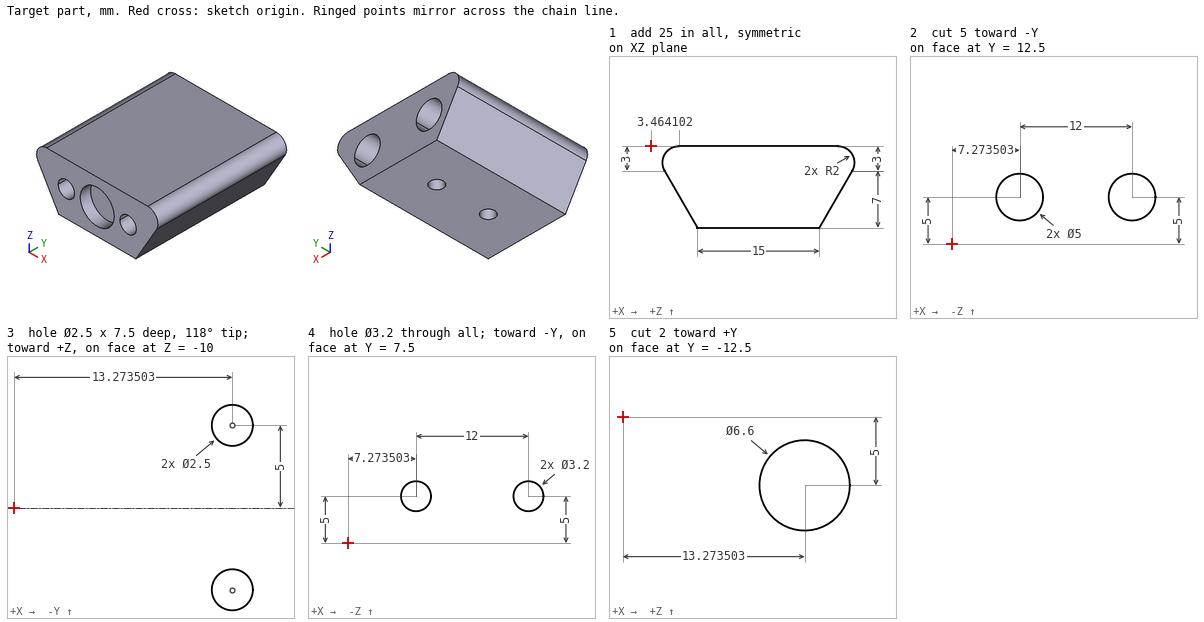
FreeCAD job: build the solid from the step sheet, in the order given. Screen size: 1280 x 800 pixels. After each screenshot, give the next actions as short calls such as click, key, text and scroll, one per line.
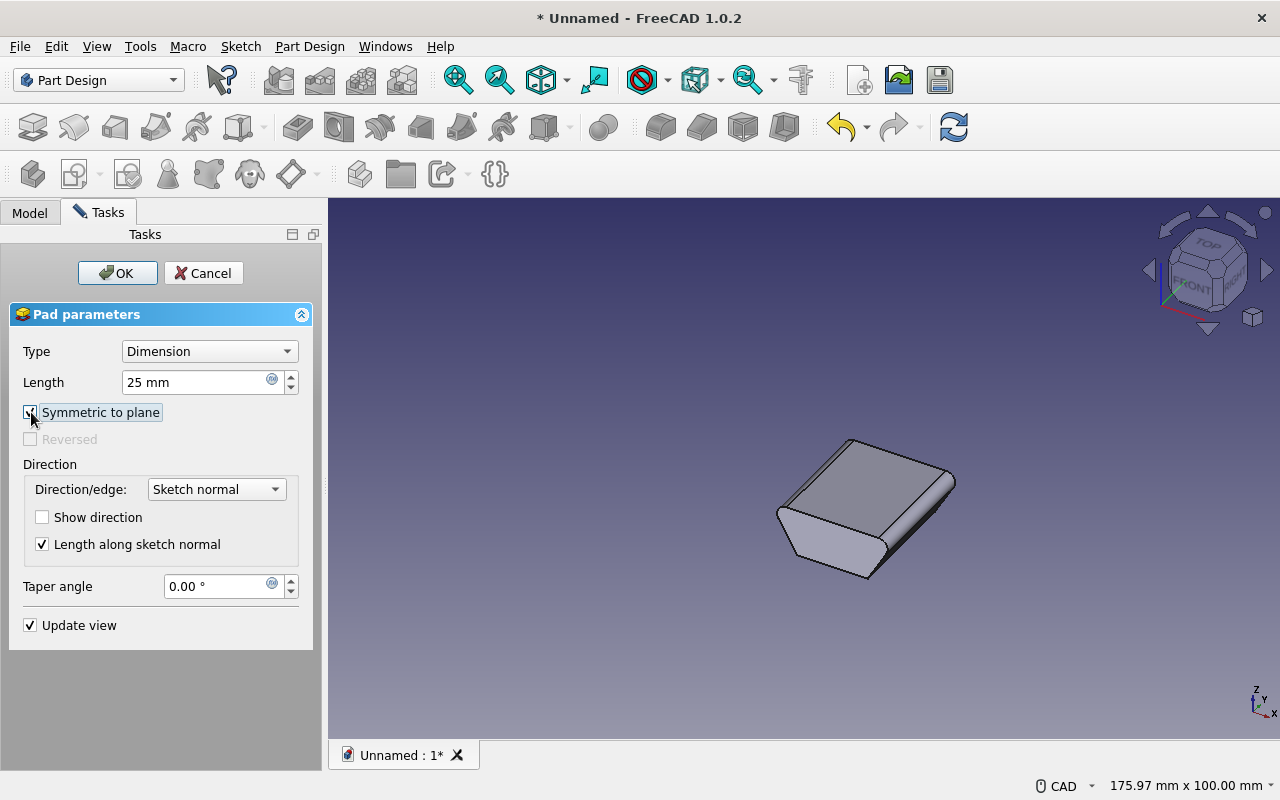
click(118, 273)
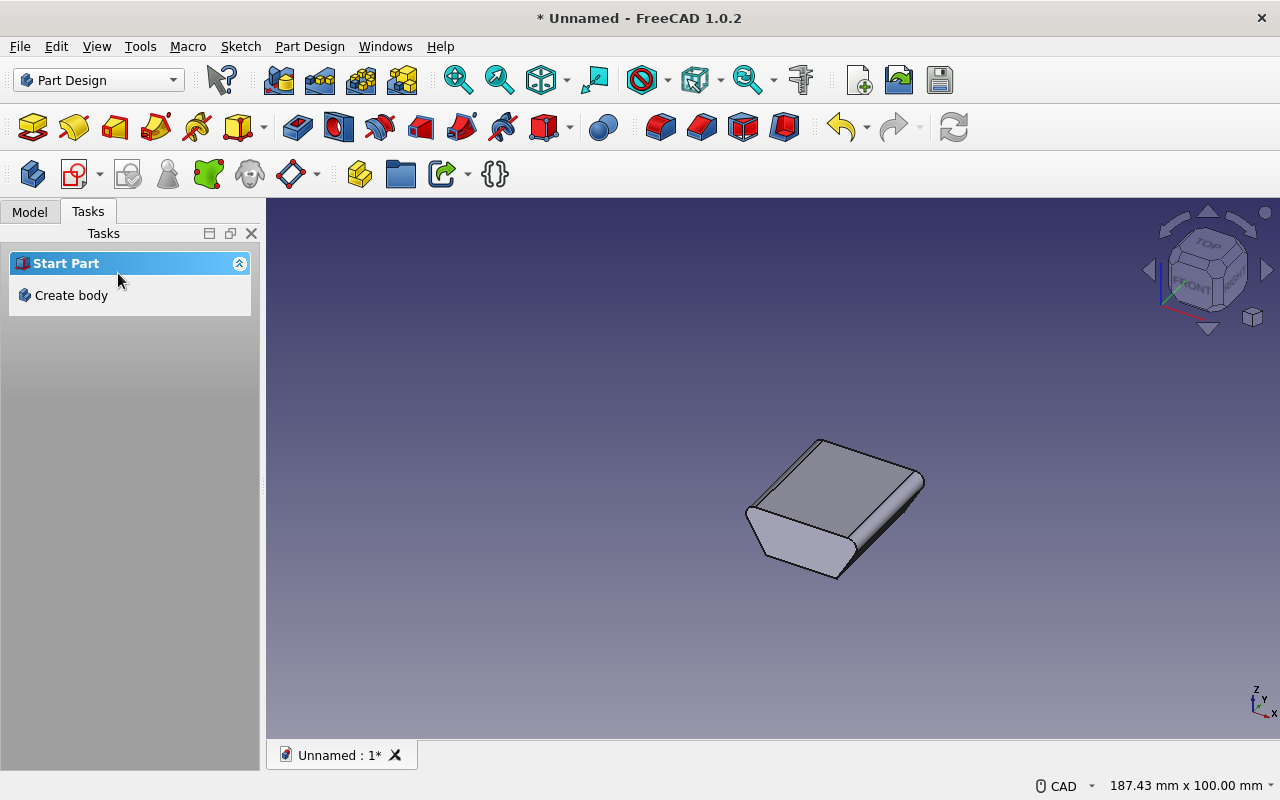
click(459, 80)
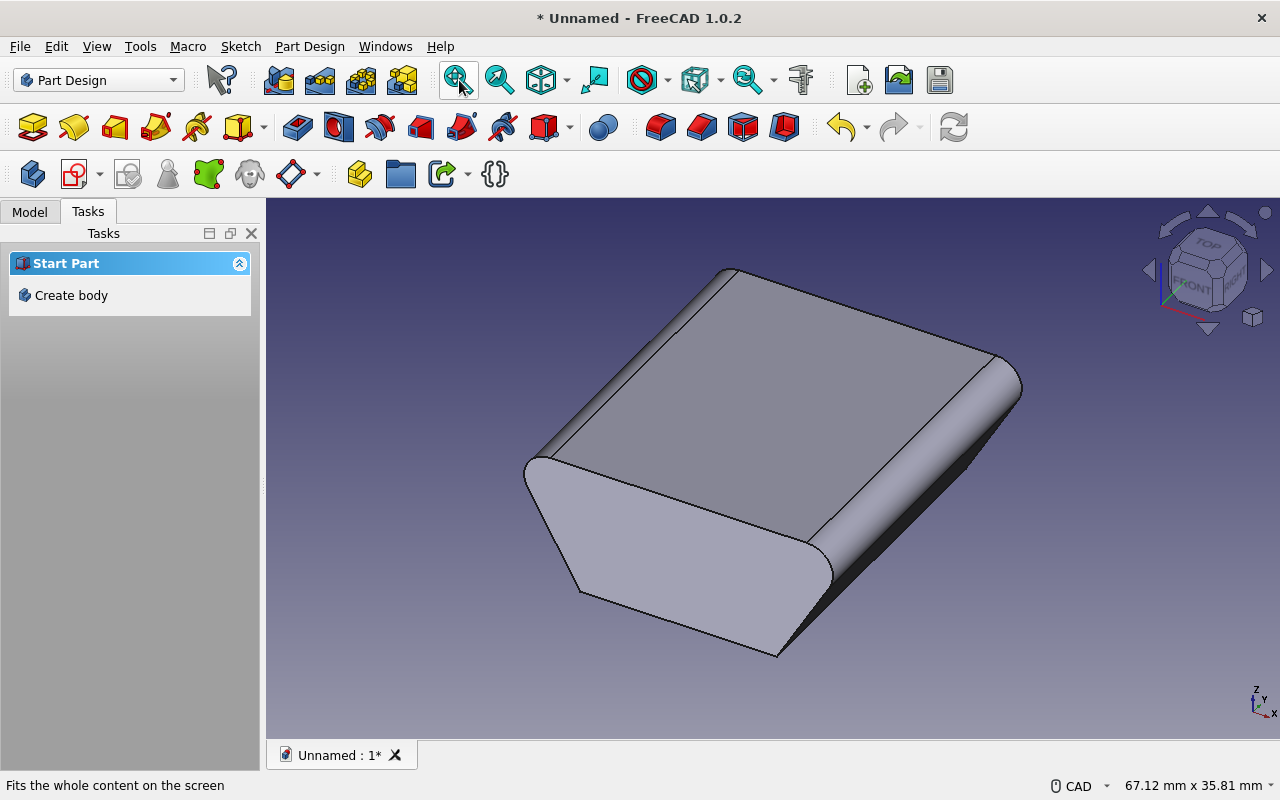
key(4)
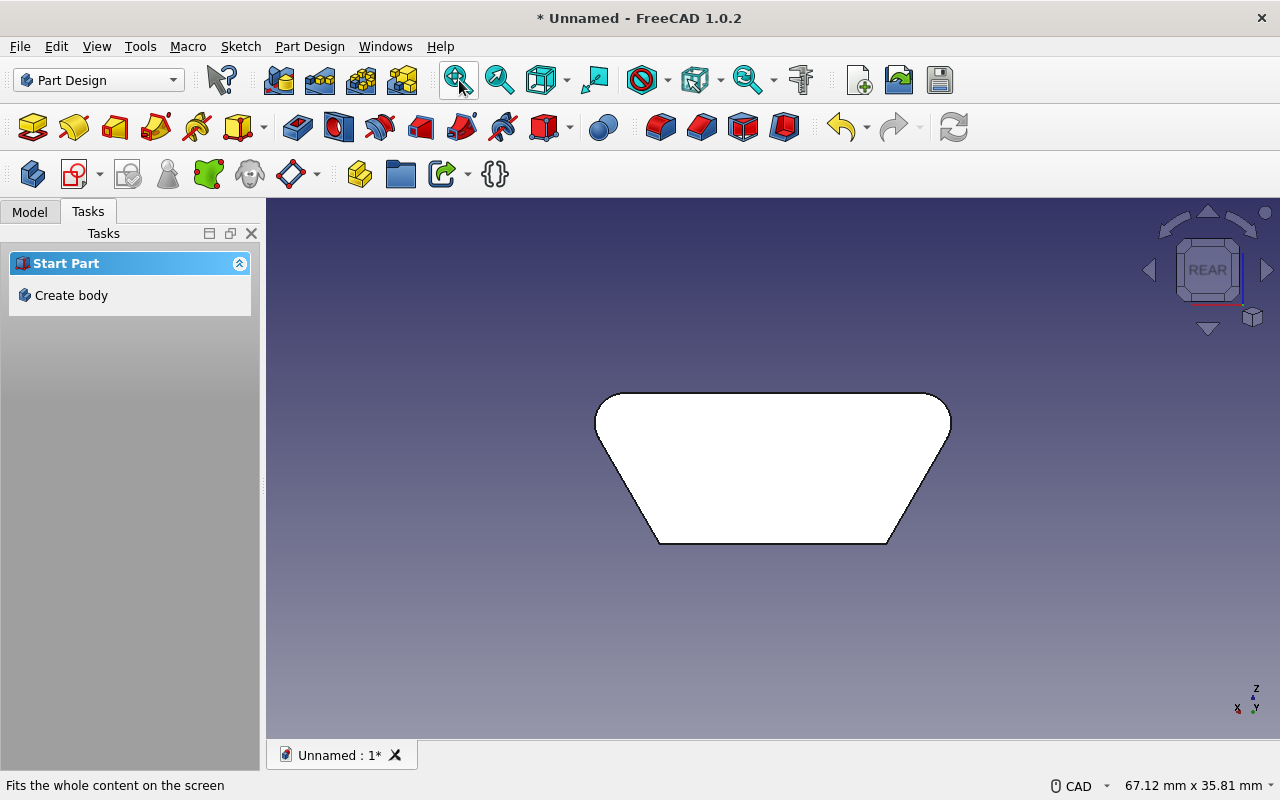
click(459, 80)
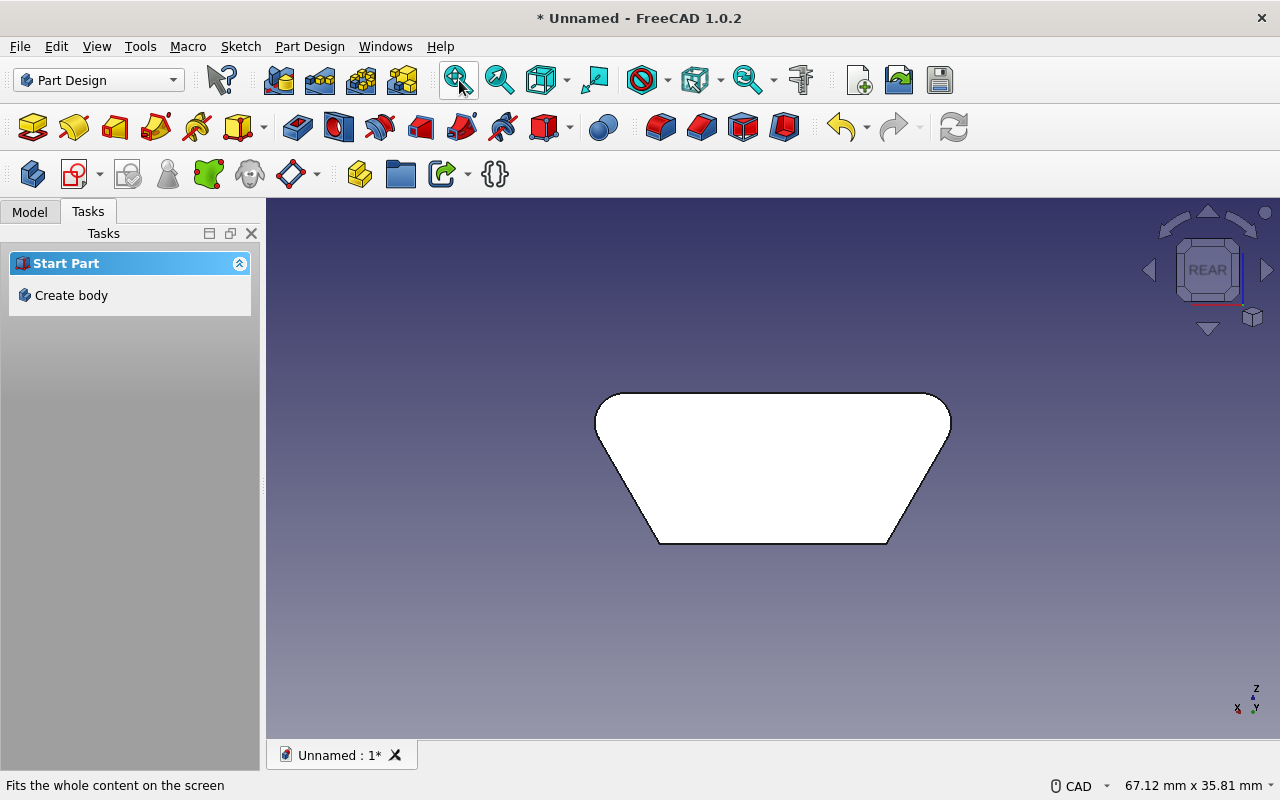
click(722, 467)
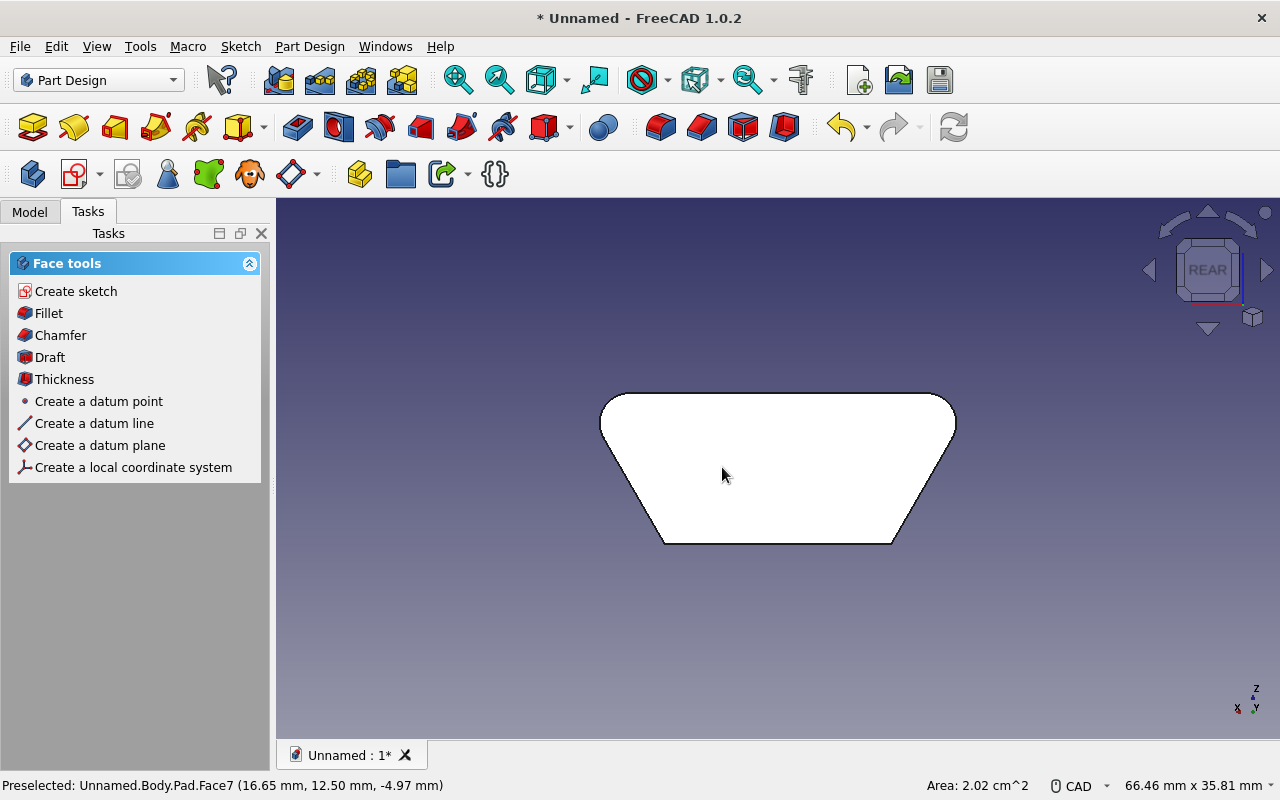
click(74, 174)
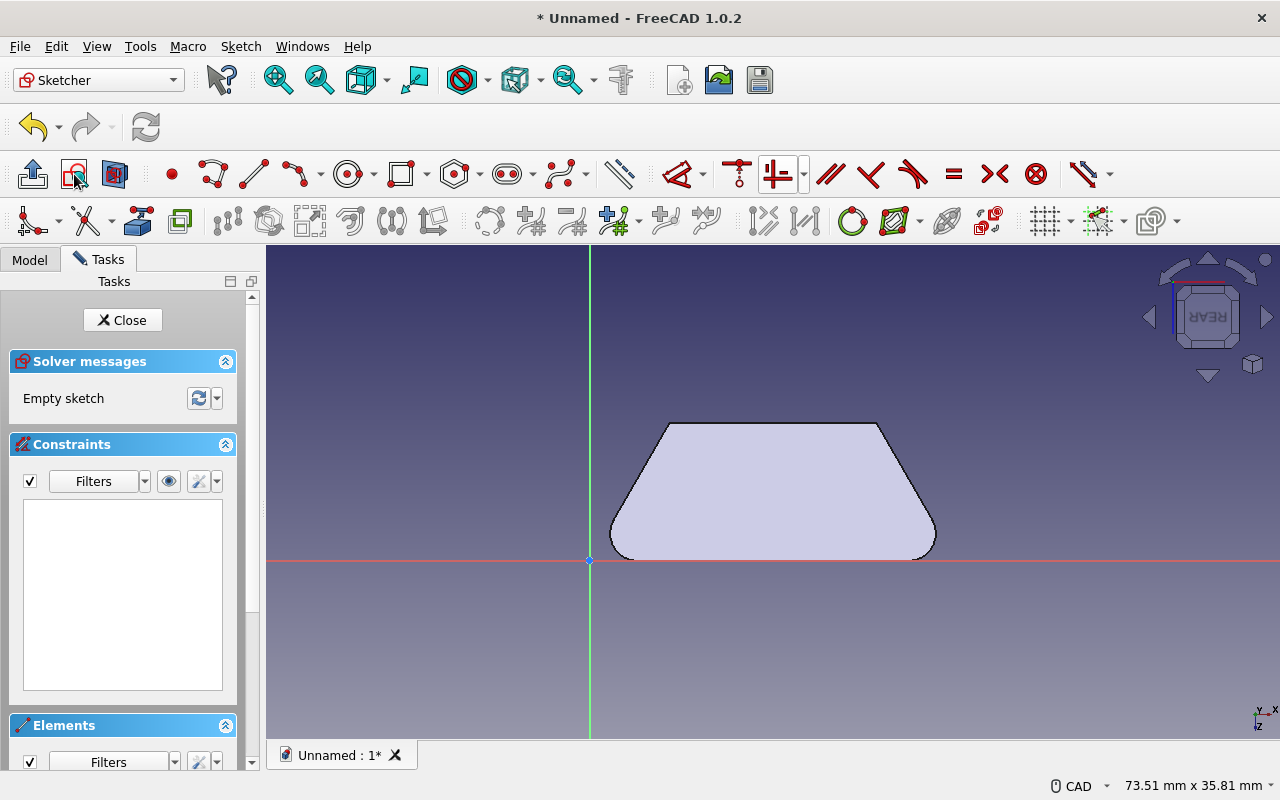
scroll(783, 530, up, 3)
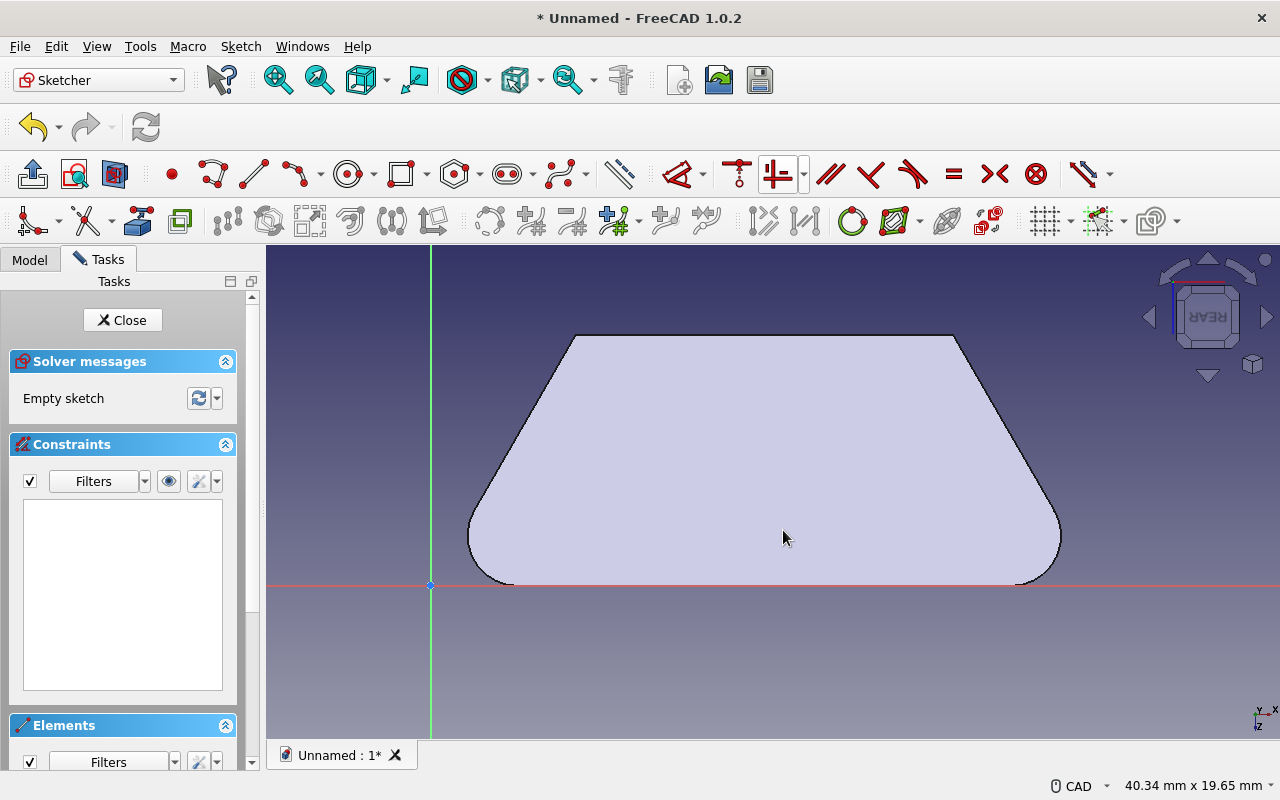
click(348, 174)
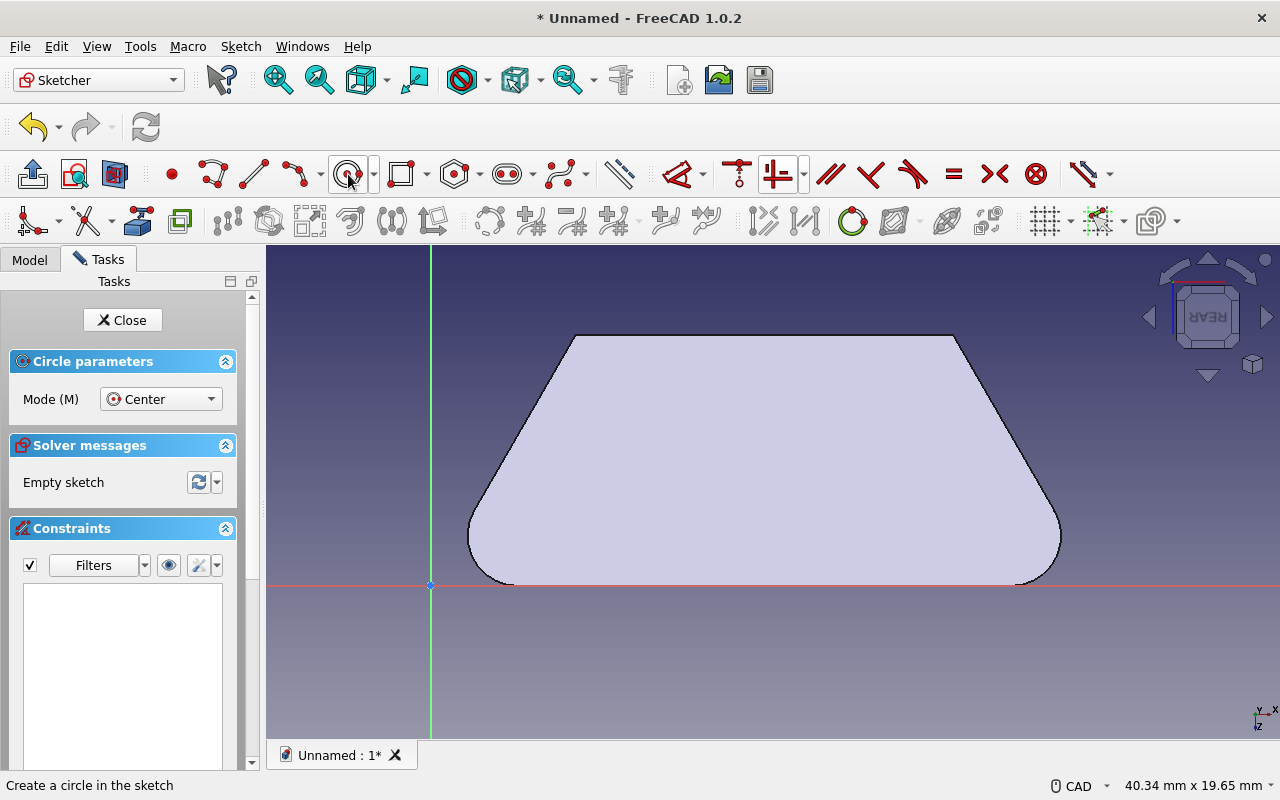
click(614, 460)
click(658, 416)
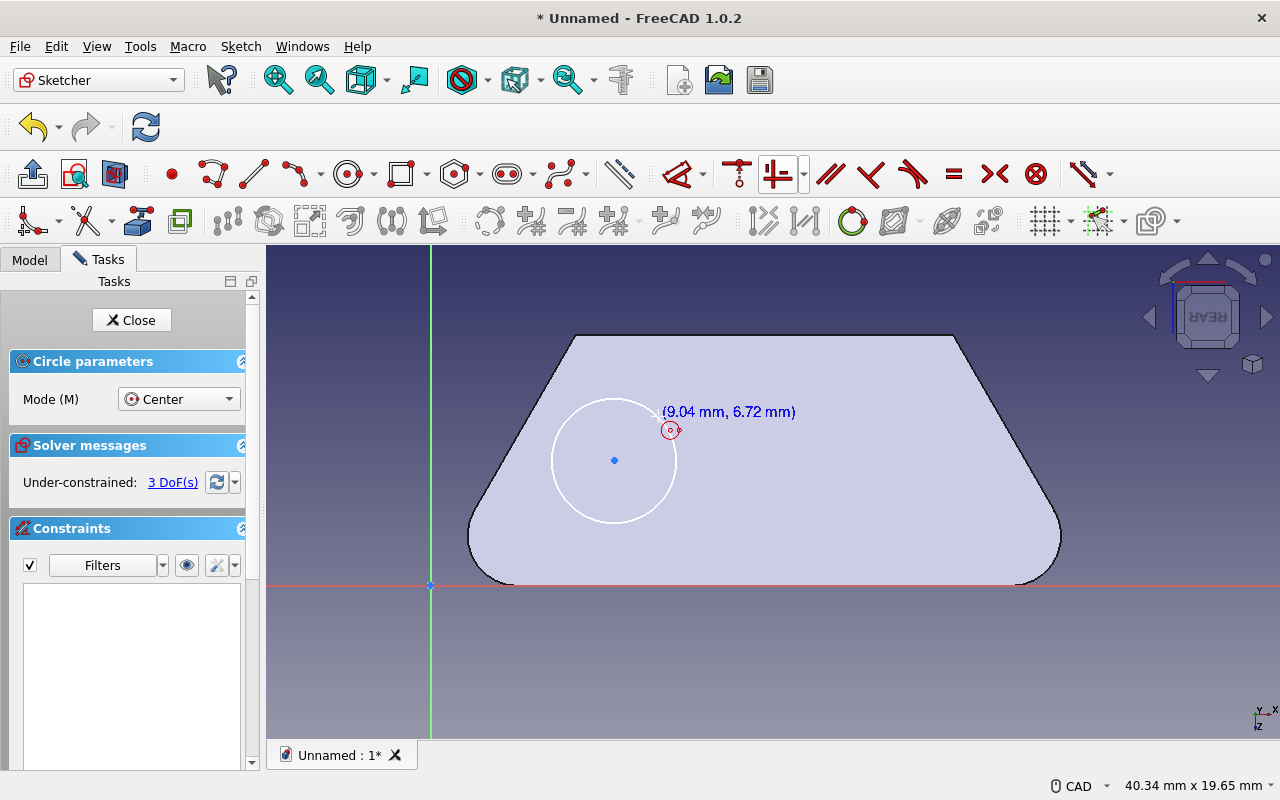
click(915, 460)
click(960, 416)
key(Escape)